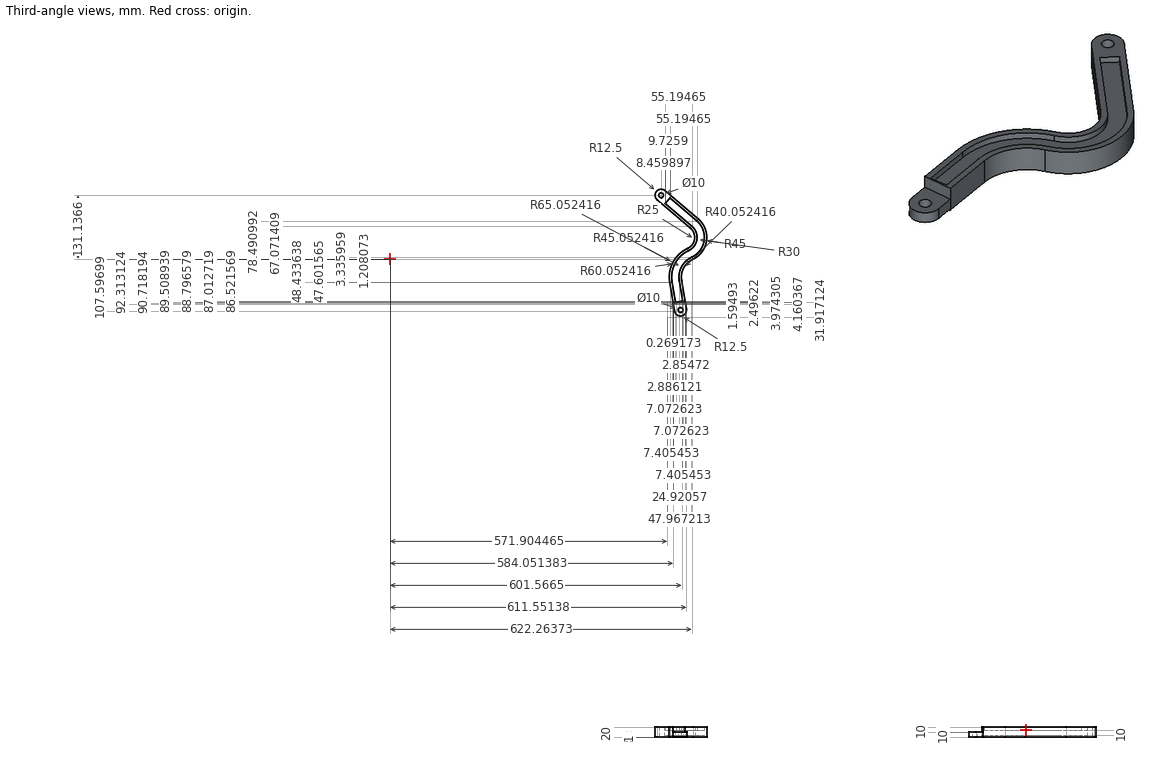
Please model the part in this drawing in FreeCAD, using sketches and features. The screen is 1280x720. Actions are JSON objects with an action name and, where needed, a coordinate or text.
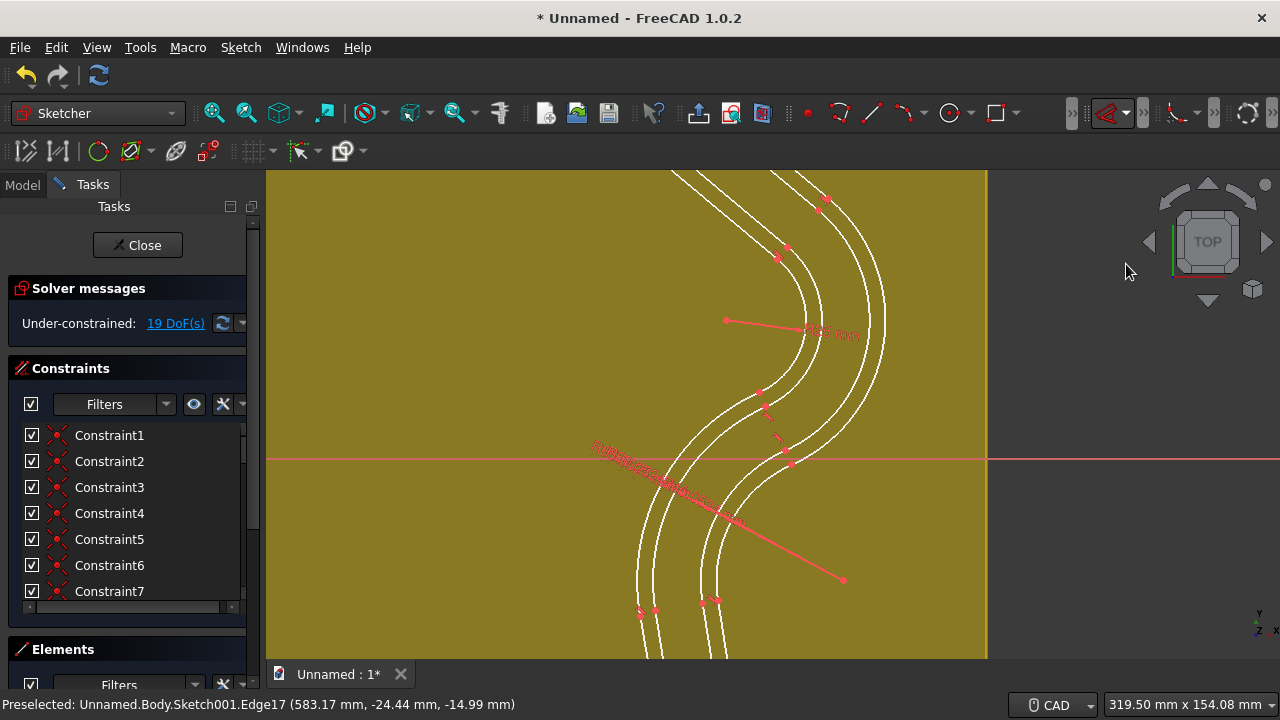
{"action": "left_click", "coordinate": [849, 394]}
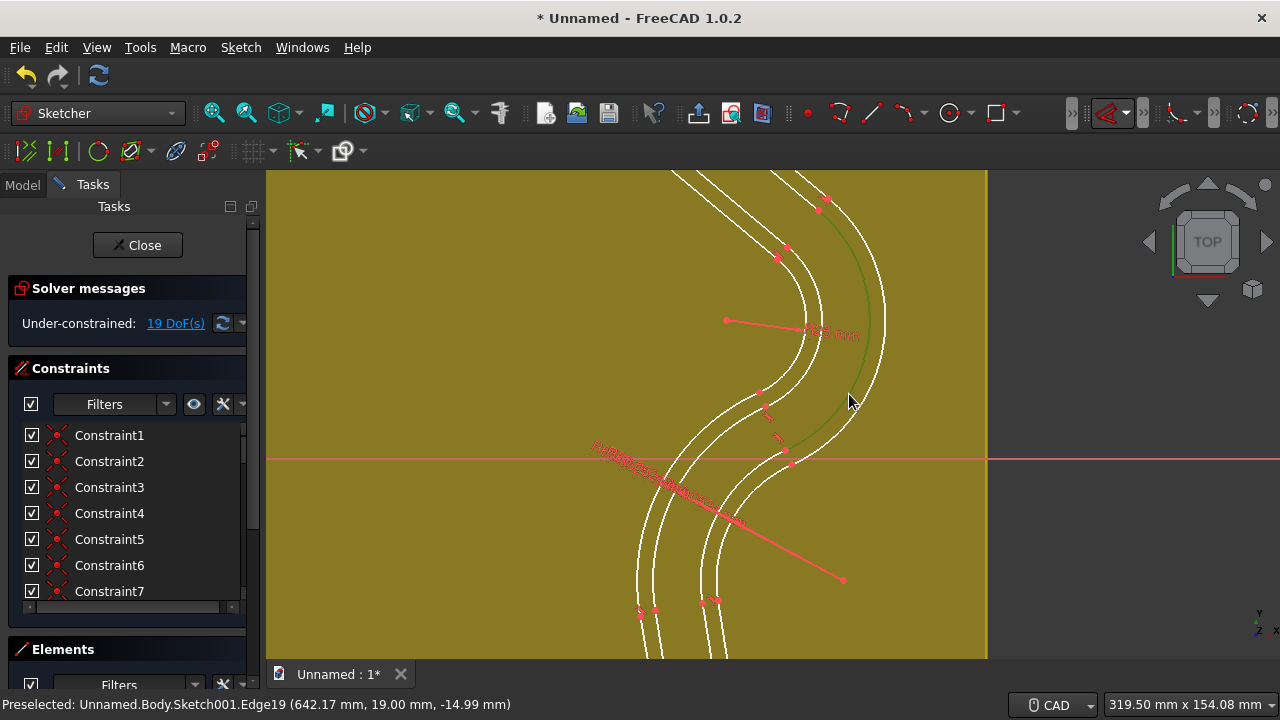
{"action": "left_click", "coordinate": [1128, 114]}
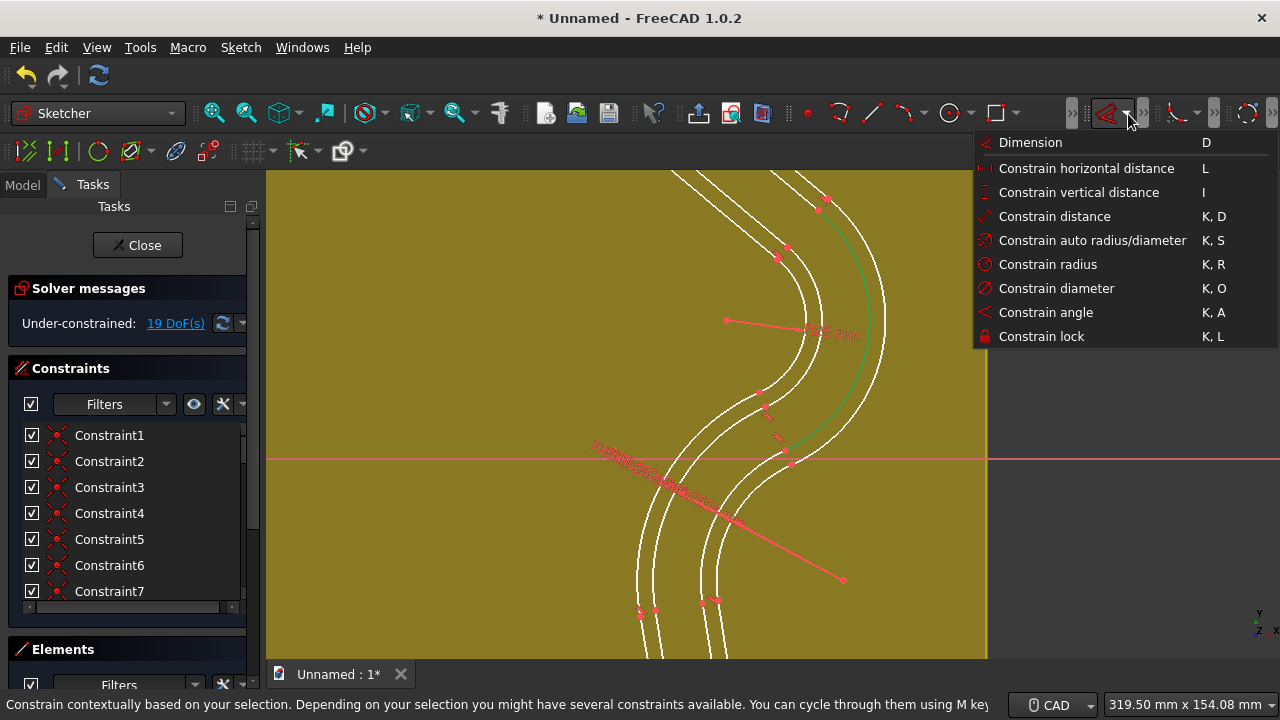
{"action": "left_click", "coordinate": [1126, 264]}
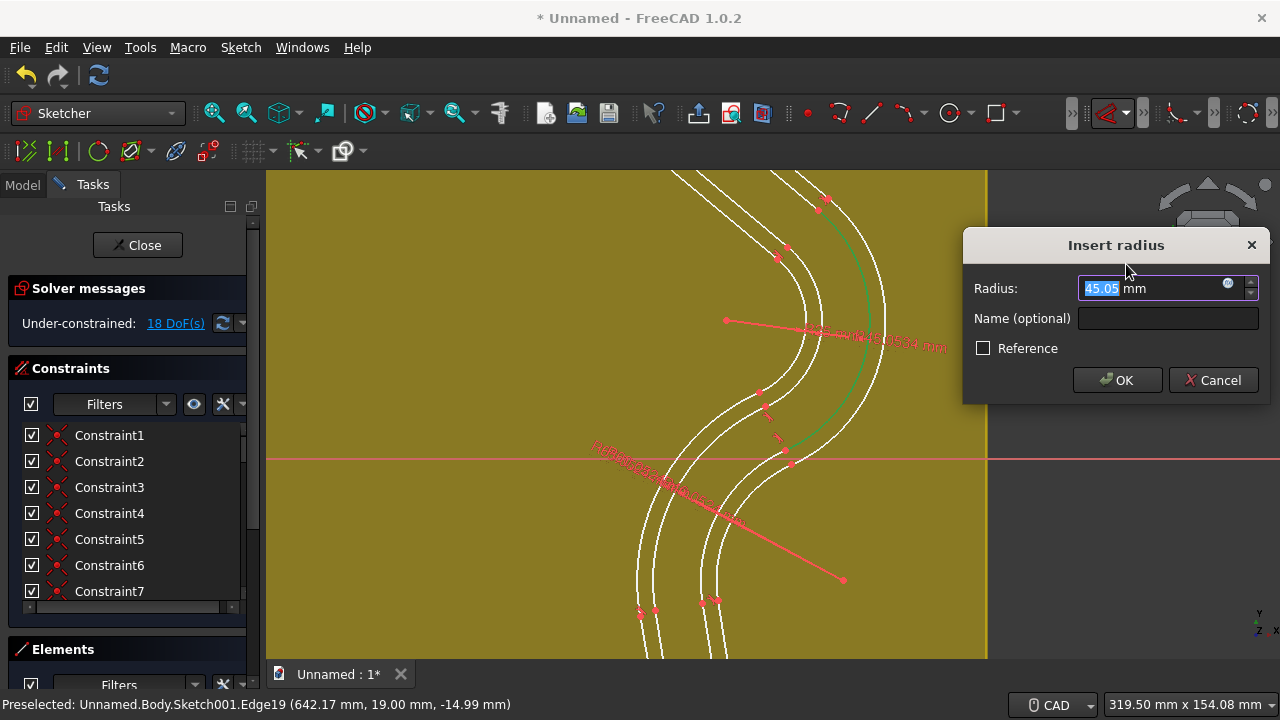
{"action": "type", "text": "45"}
{"action": "key", "text": "Return"}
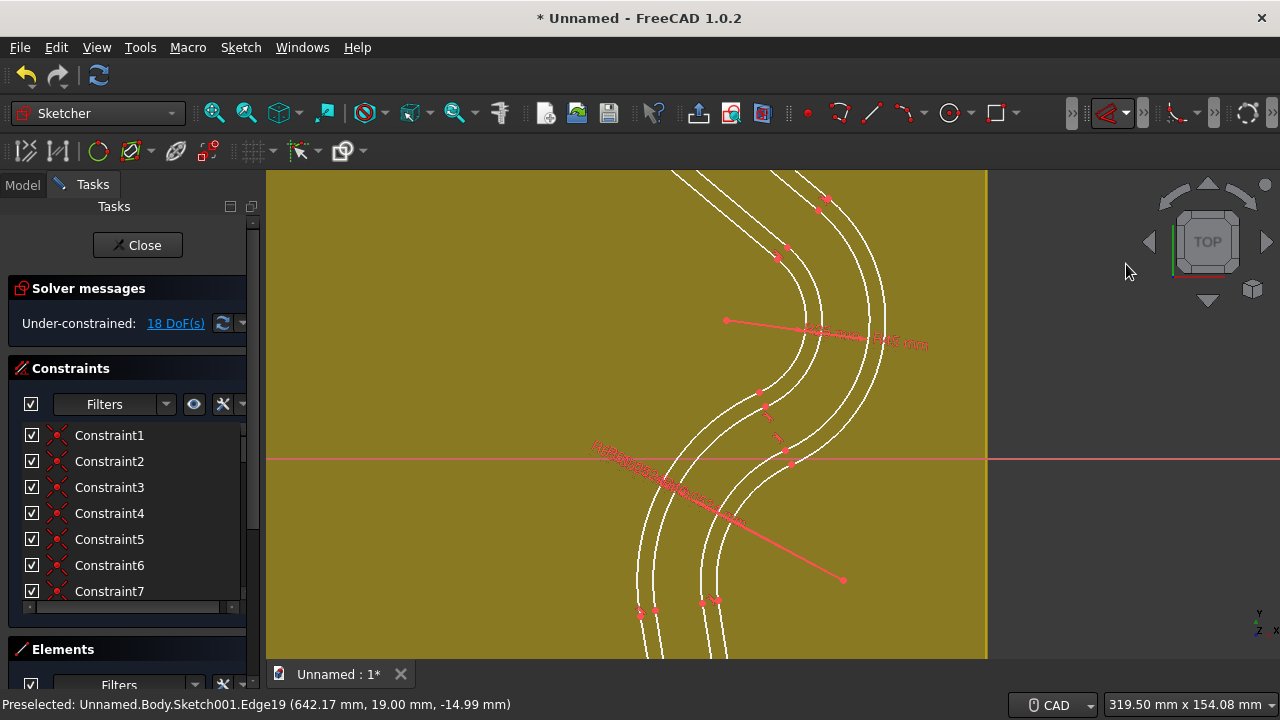
{"action": "scroll", "coordinate": [695, 441], "scroll_direction": "down", "scroll_amount": 4}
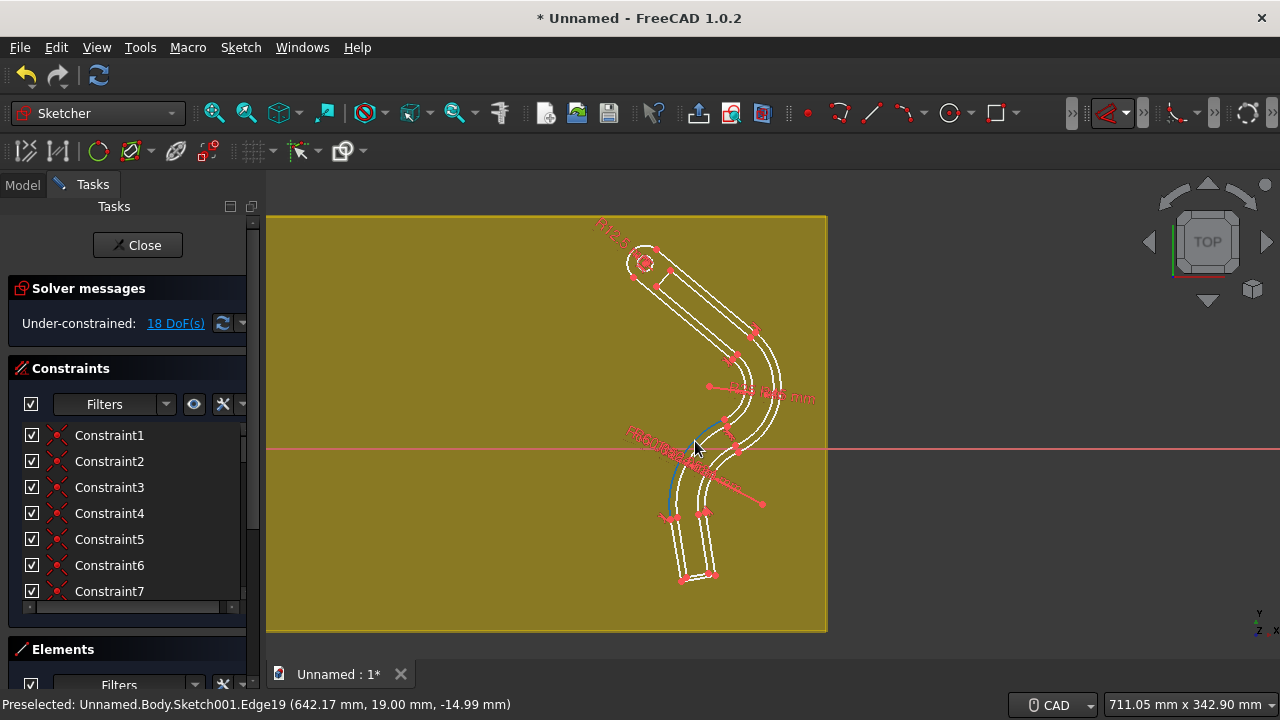
{"action": "scroll", "coordinate": [651, 258], "scroll_direction": "up", "scroll_amount": 6}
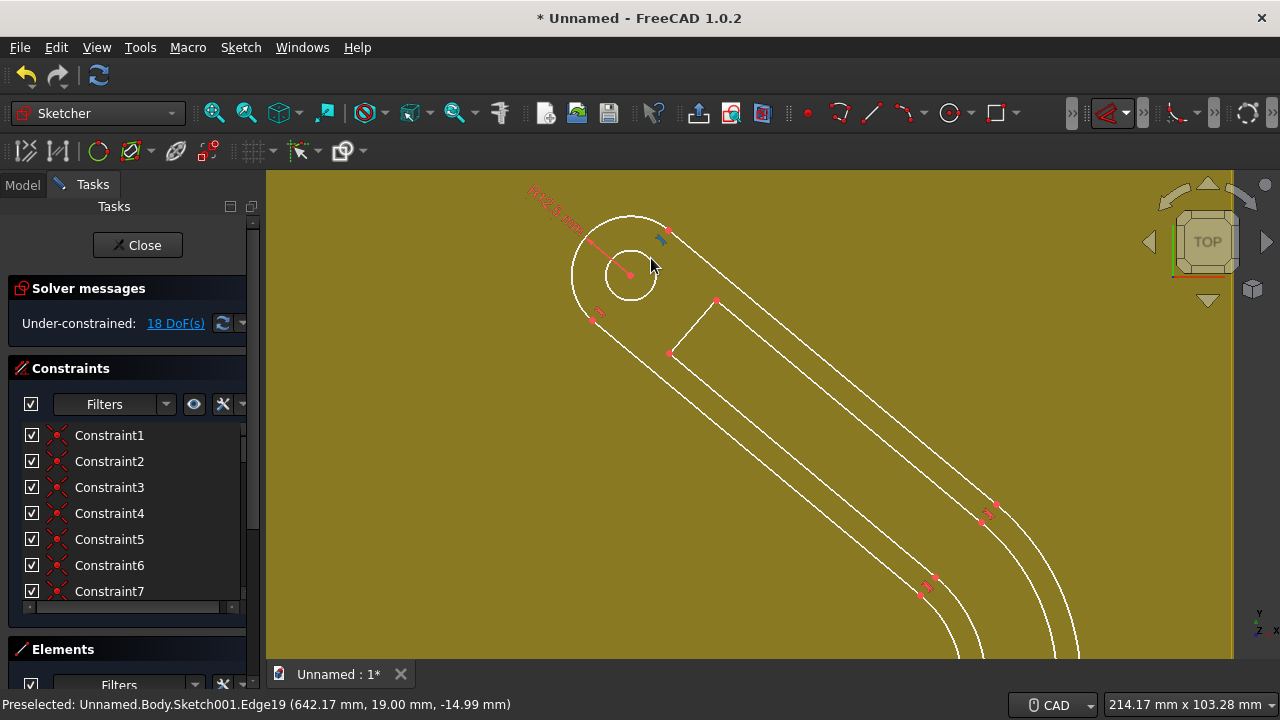
{"action": "left_click", "coordinate": [648, 258]}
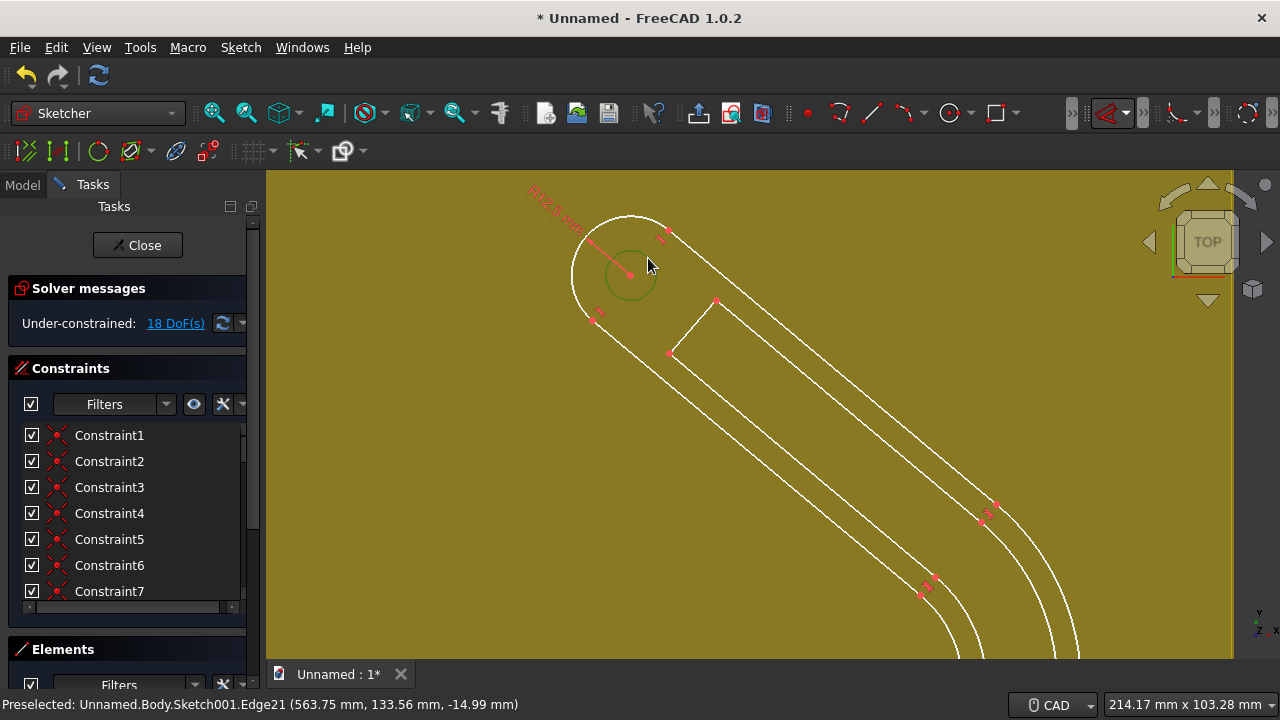
{"action": "left_click", "coordinate": [1128, 114]}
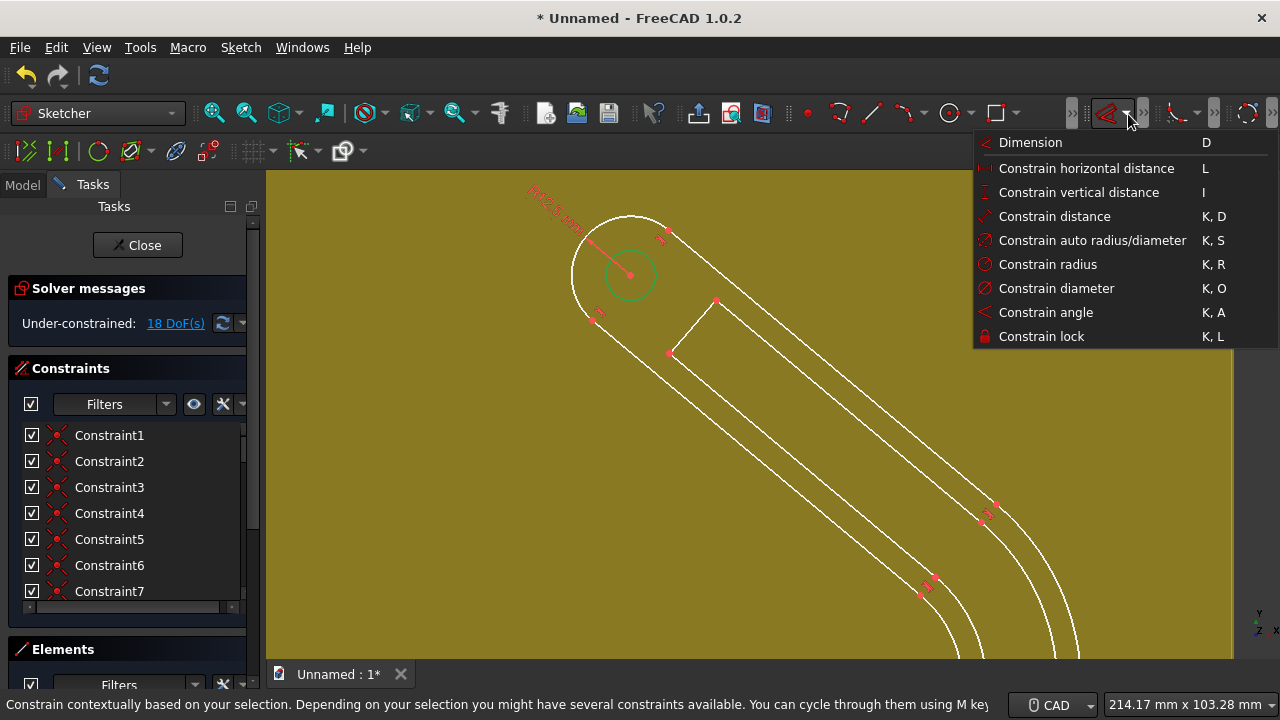
{"action": "left_click", "coordinate": [1126, 288]}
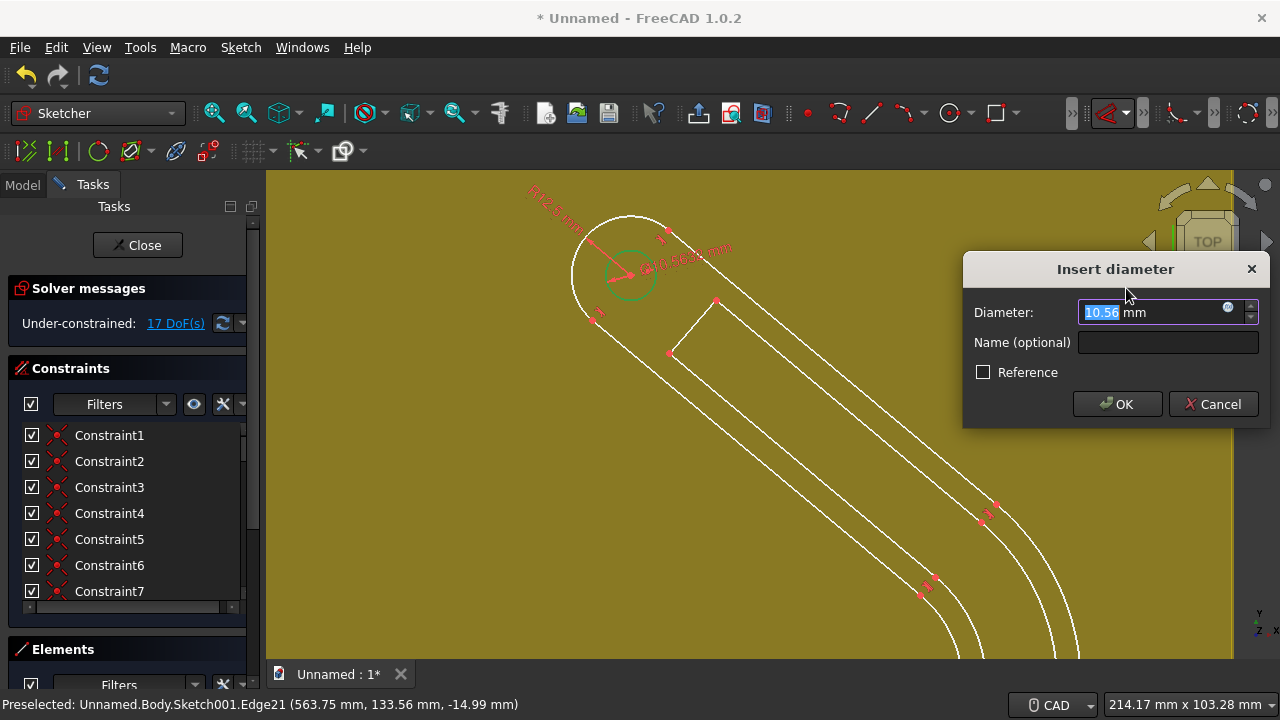
{"action": "type", "text": "10"}
{"action": "key", "text": "Return"}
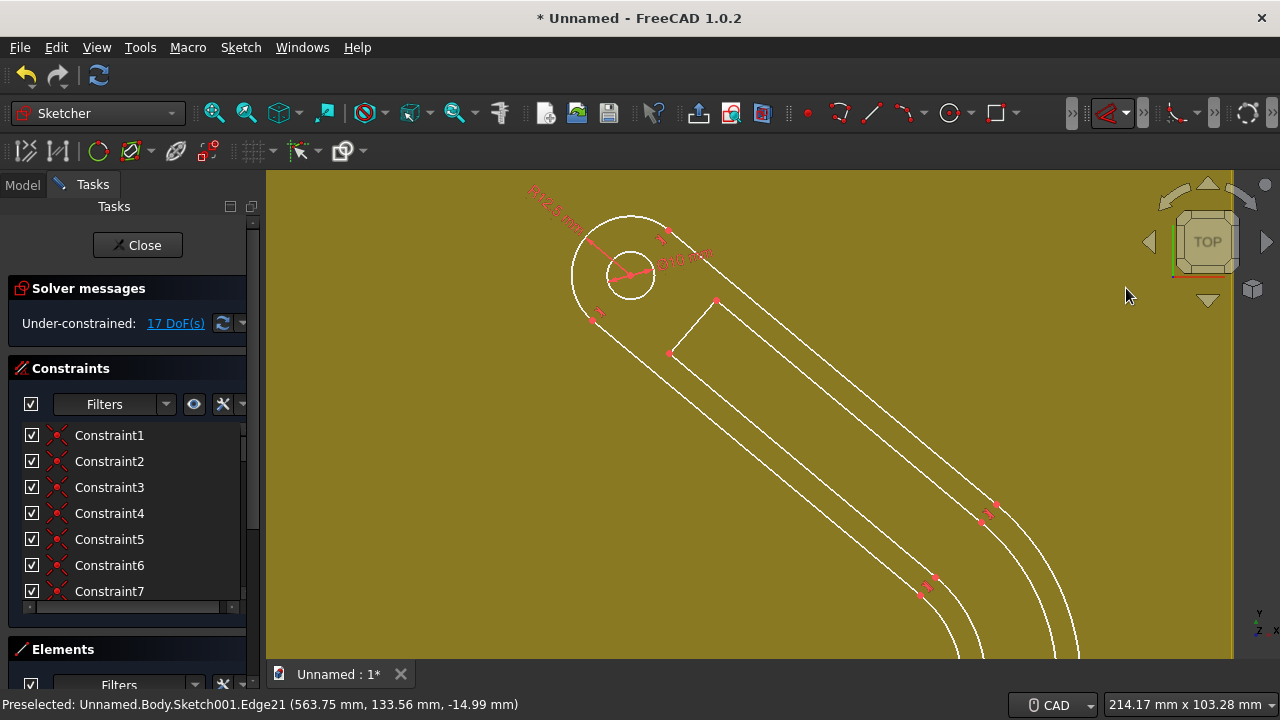
{"action": "left_click", "coordinate": [684, 338]}